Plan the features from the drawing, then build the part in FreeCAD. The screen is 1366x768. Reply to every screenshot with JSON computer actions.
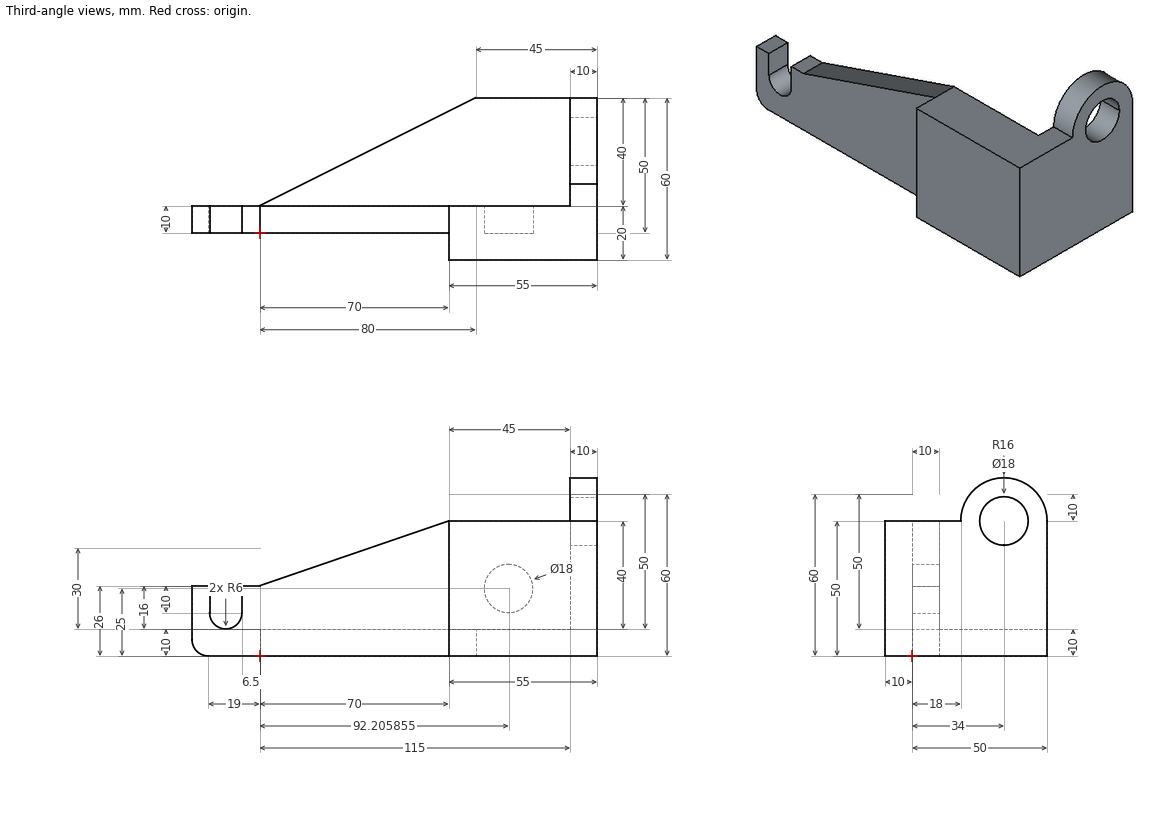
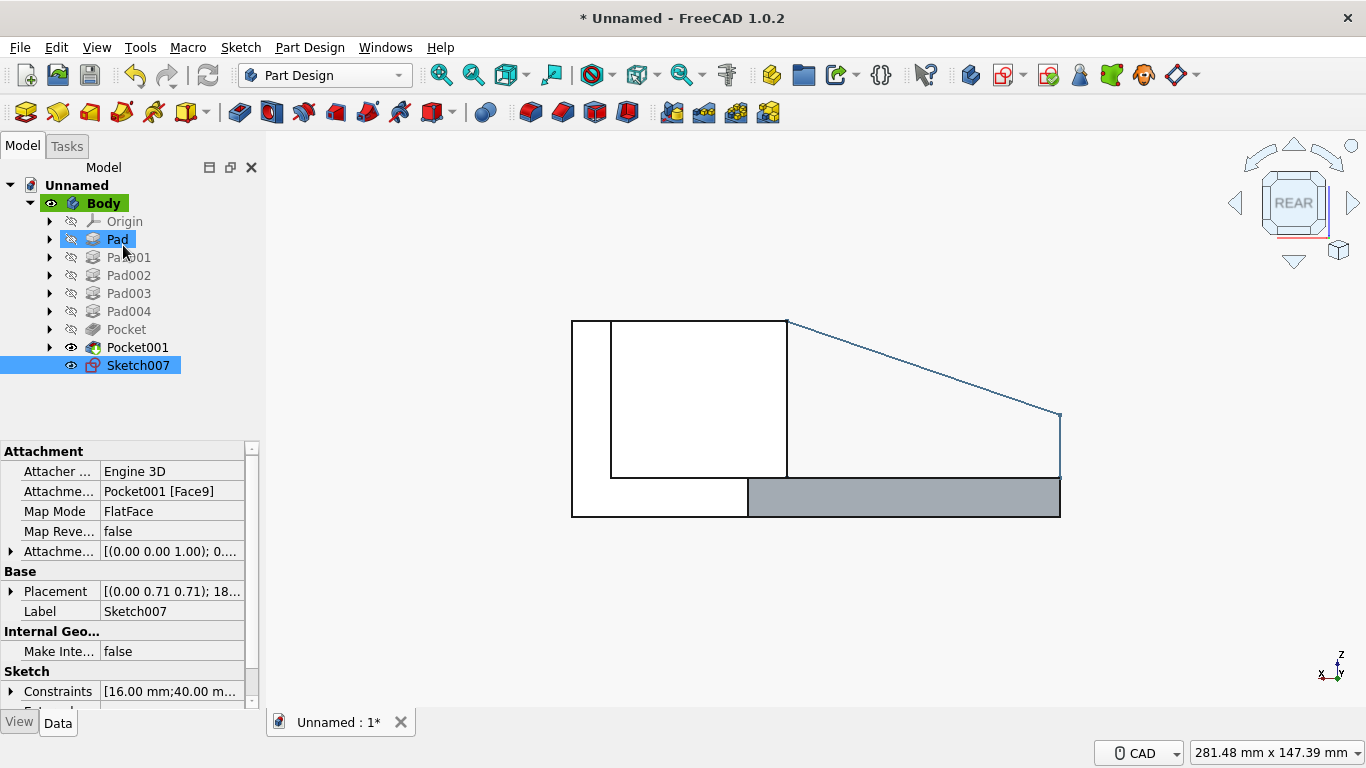
{"action": "left_click", "coordinate": [26, 112]}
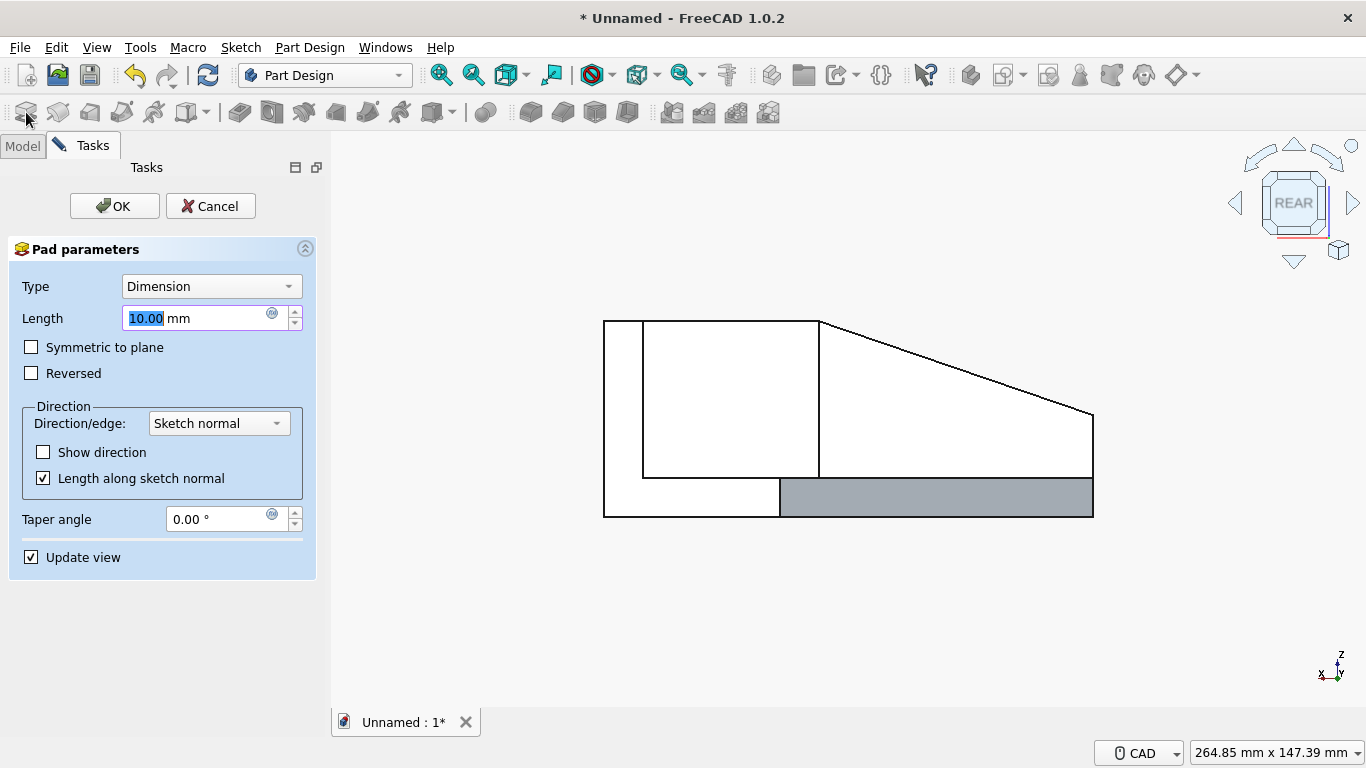
{"action": "type", "text": "10"}
{"action": "key", "text": "Tab"}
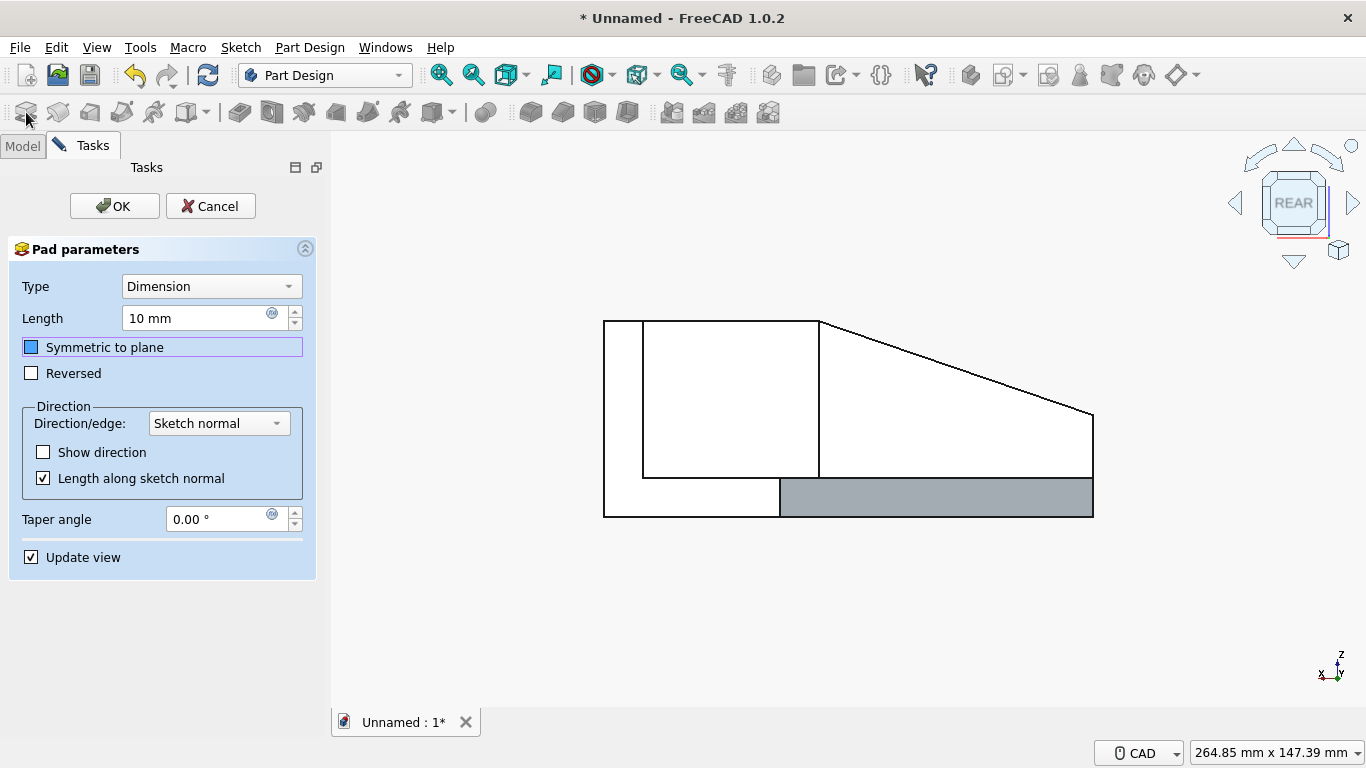
{"action": "left_click", "coordinate": [30, 373]}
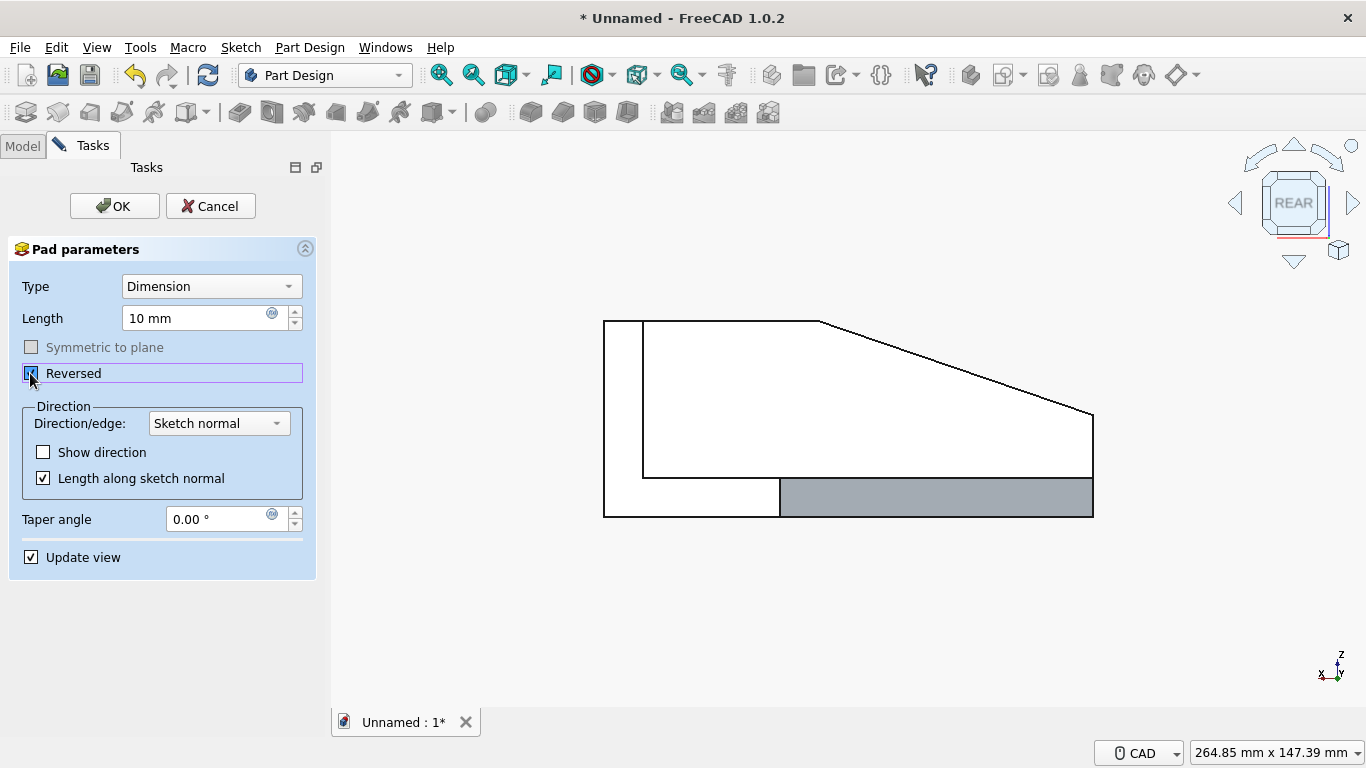
{"action": "left_click", "coordinate": [115, 206]}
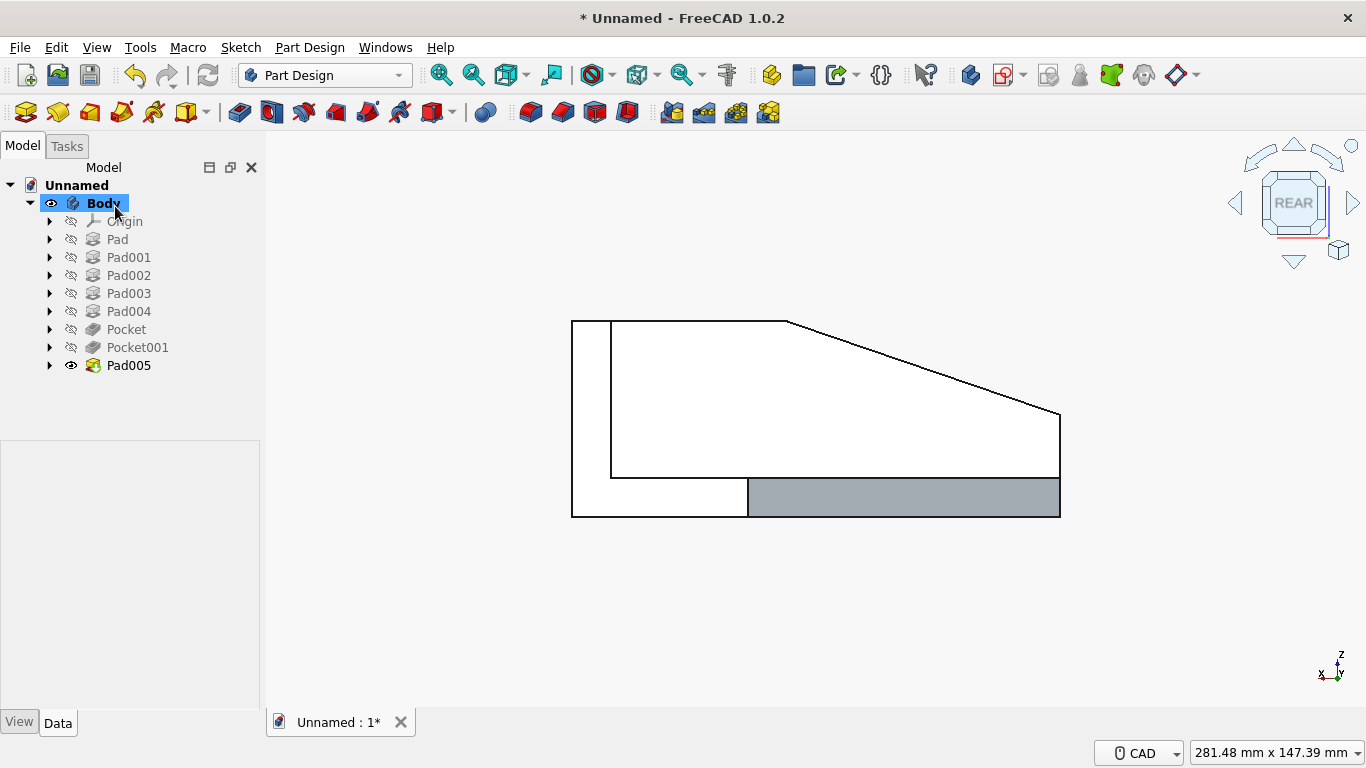
{"action": "left_click", "coordinate": [442, 76]}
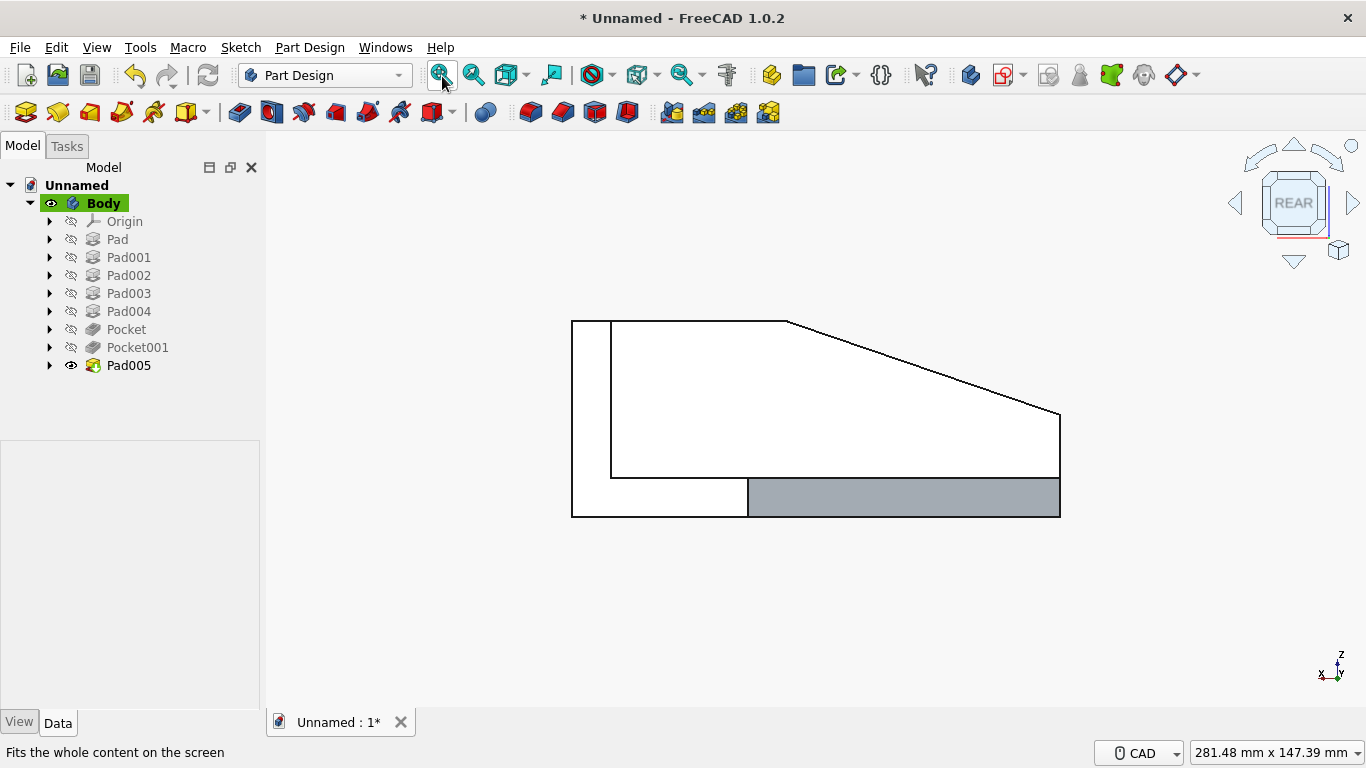
{"action": "left_click", "coordinate": [1004, 76]}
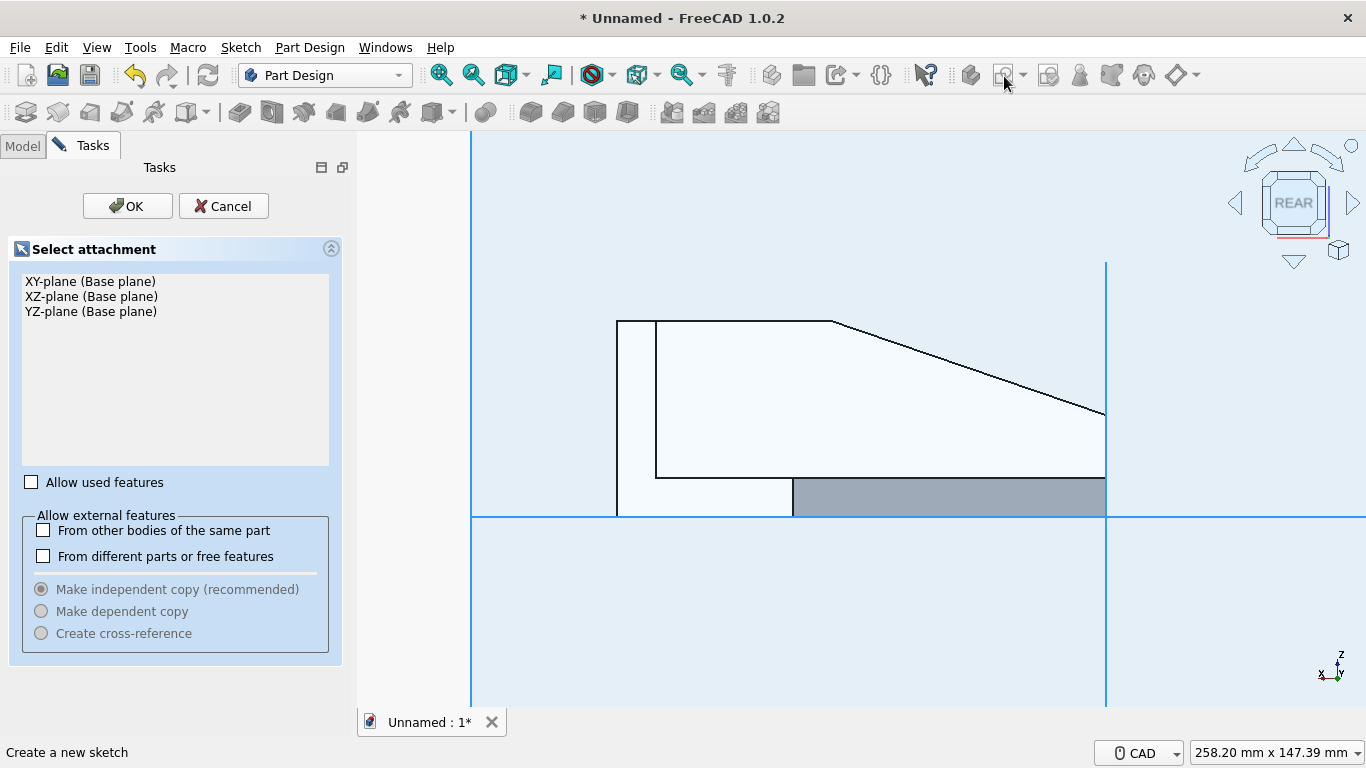
{"action": "left_click", "coordinate": [82, 296]}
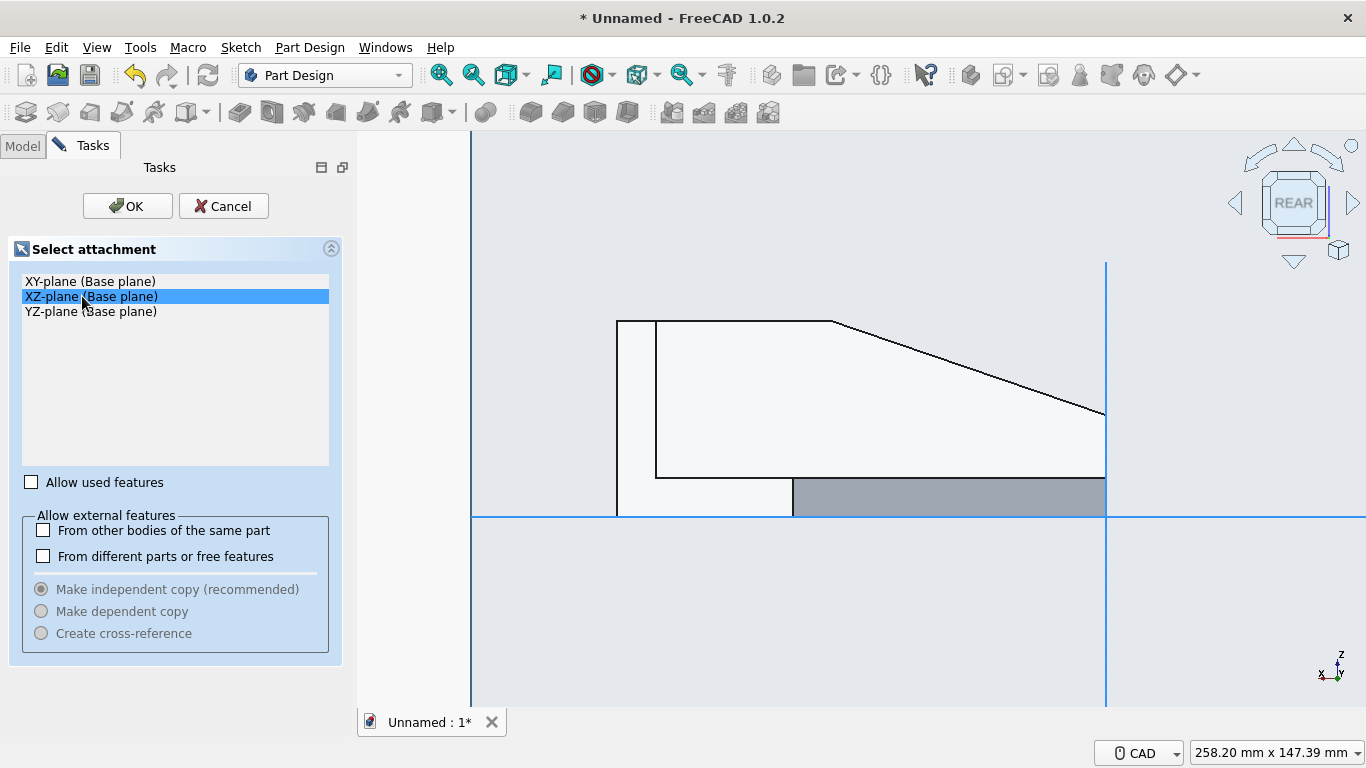
{"action": "left_click", "coordinate": [128, 206]}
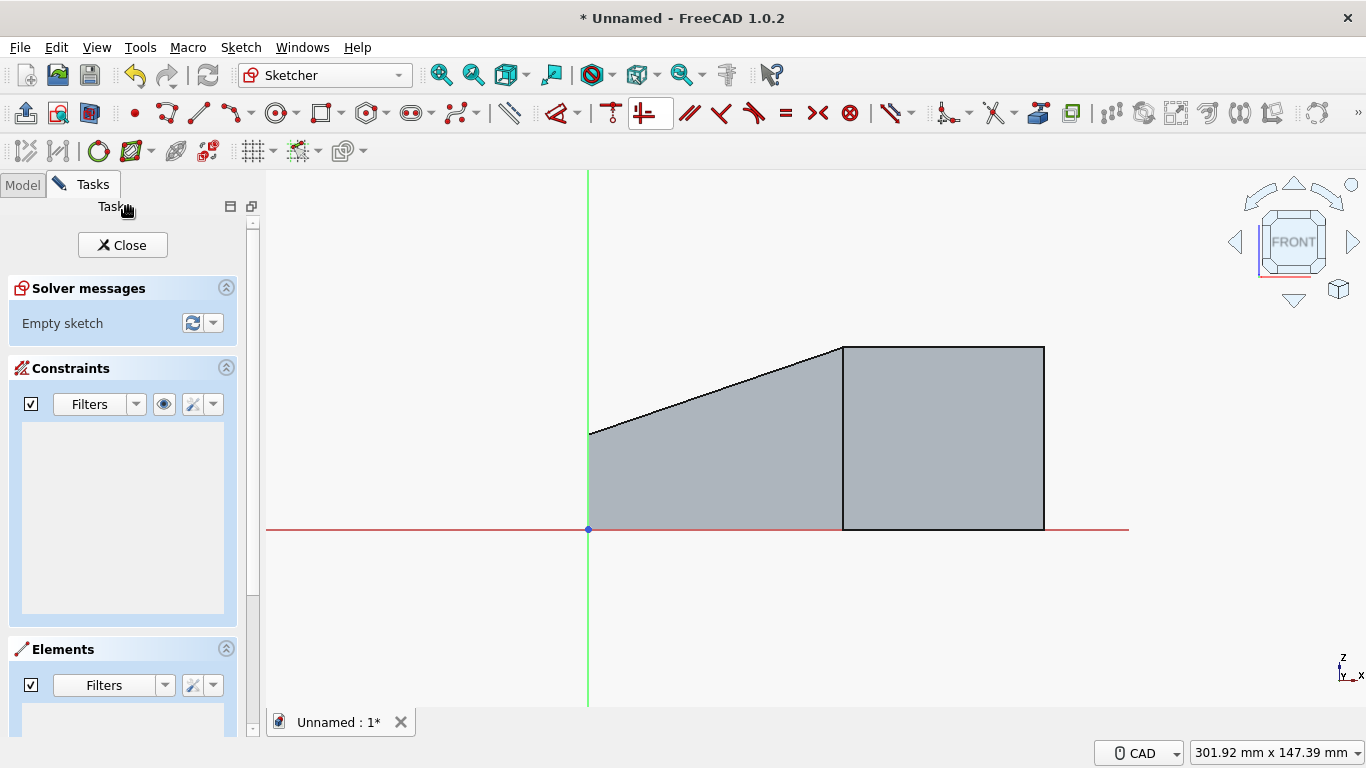
{"action": "left_click", "coordinate": [90, 114]}